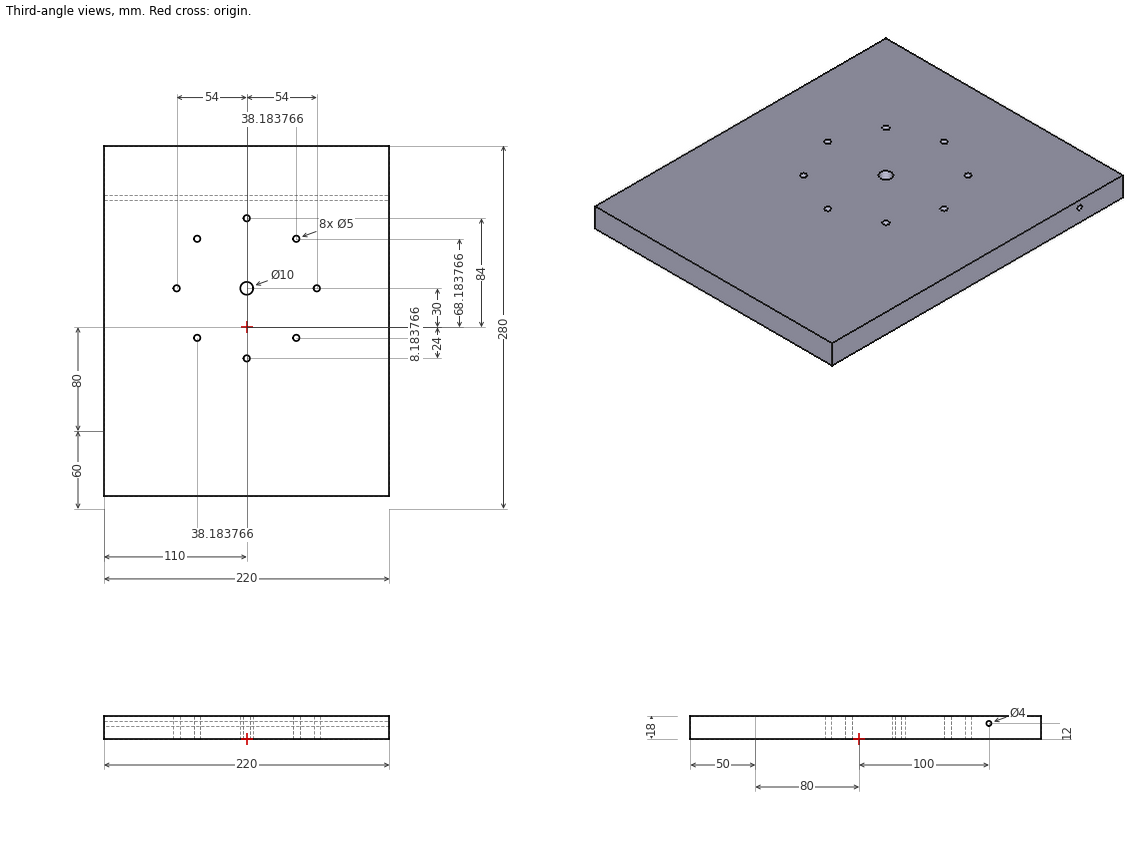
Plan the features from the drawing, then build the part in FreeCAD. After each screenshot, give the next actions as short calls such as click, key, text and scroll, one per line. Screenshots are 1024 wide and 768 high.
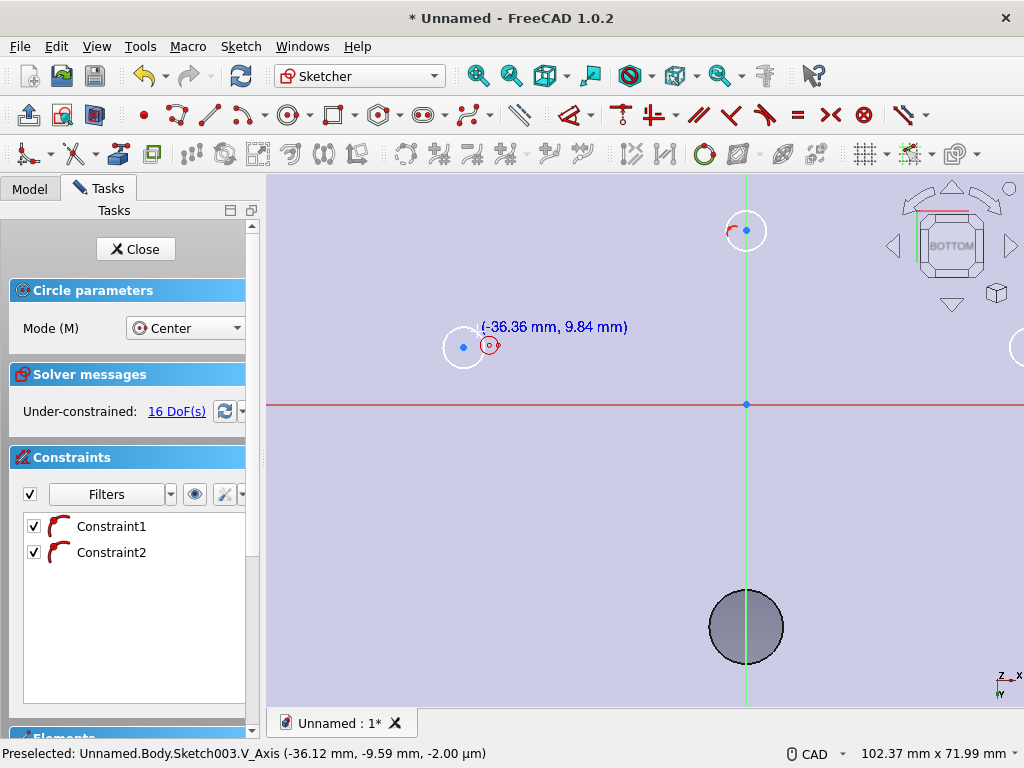
scroll(346, 627, up, 2)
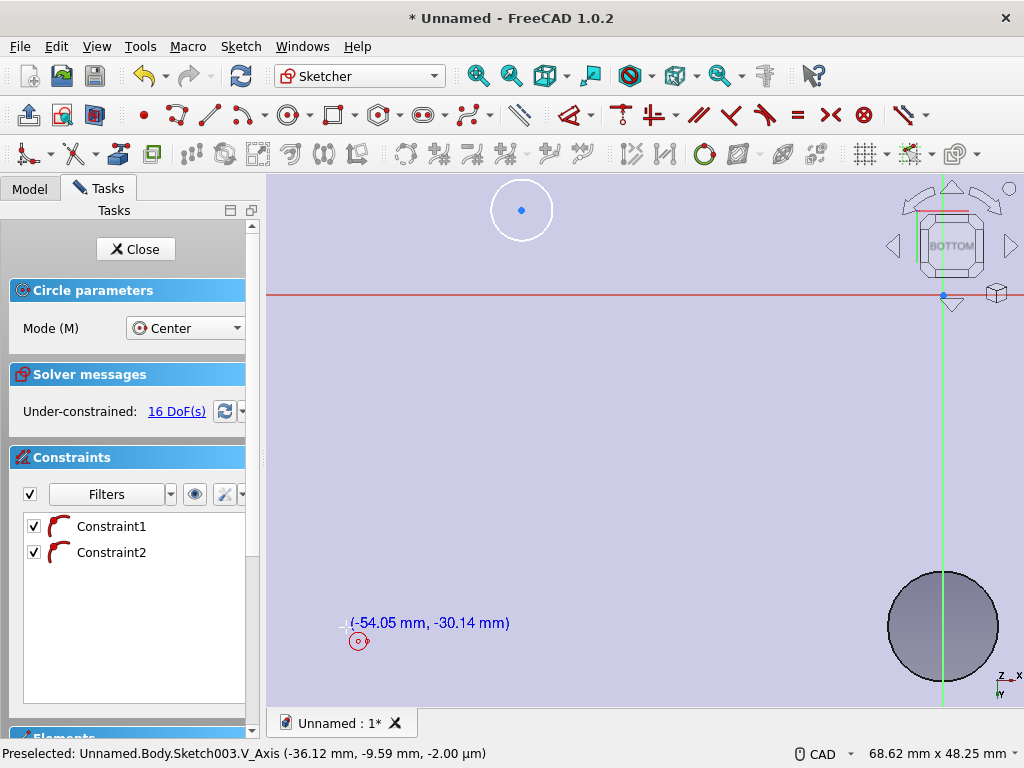
scroll(457, 380, down, 7)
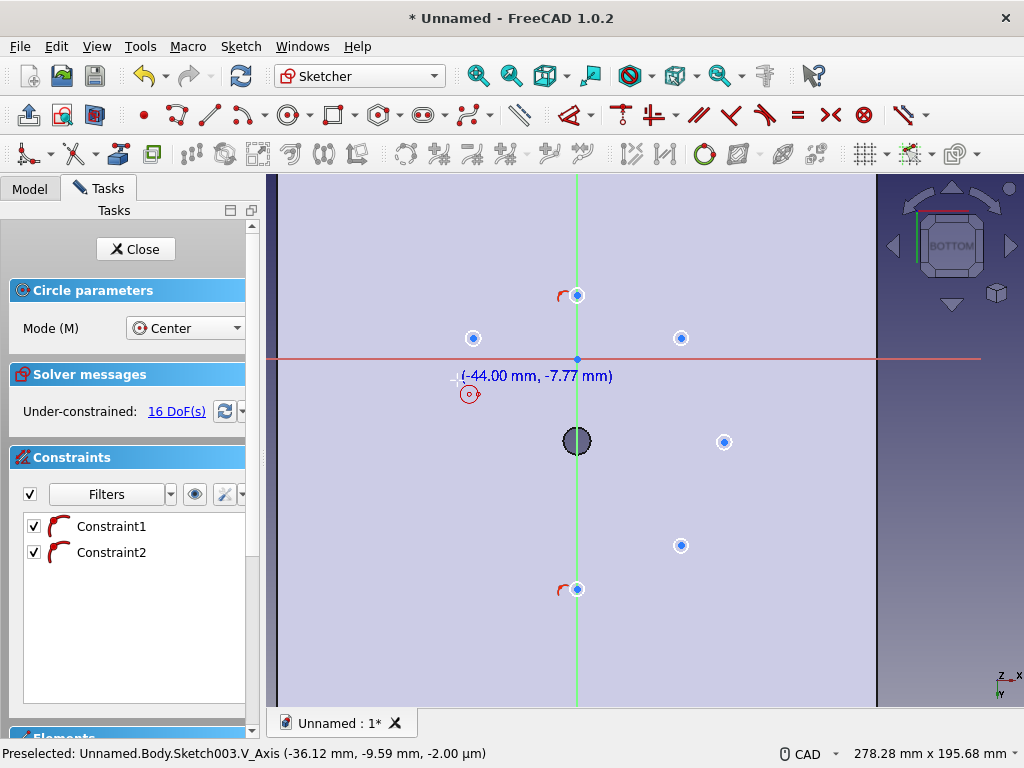
click(430, 441)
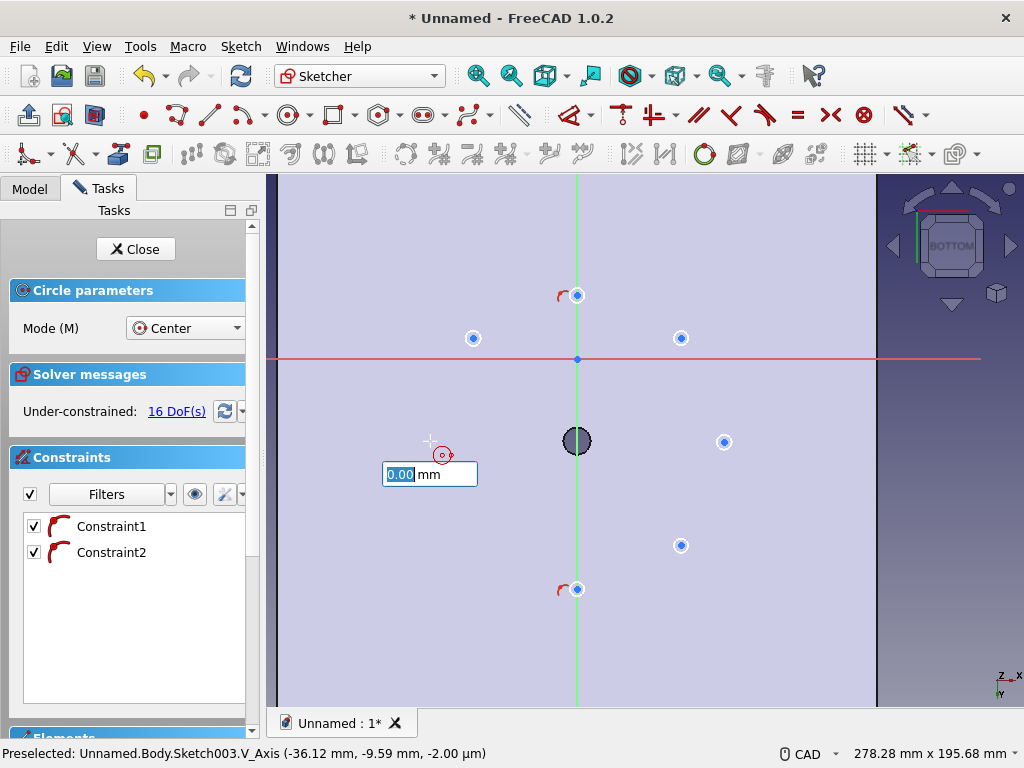
scroll(435, 436, up, 5)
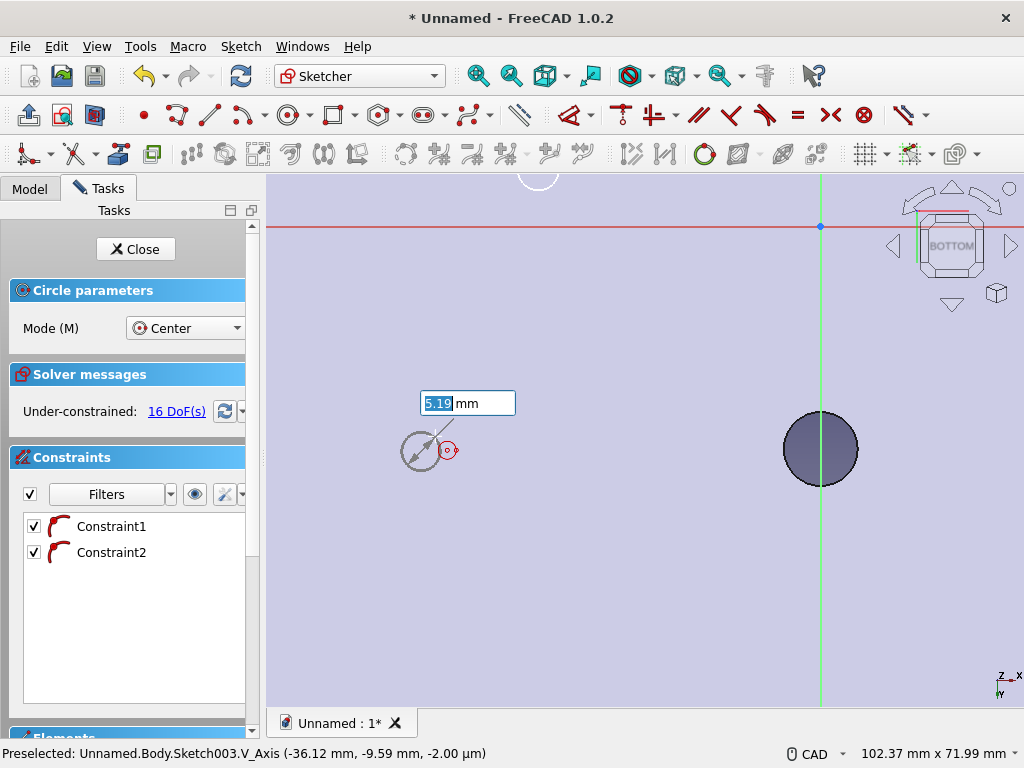
click(434, 436)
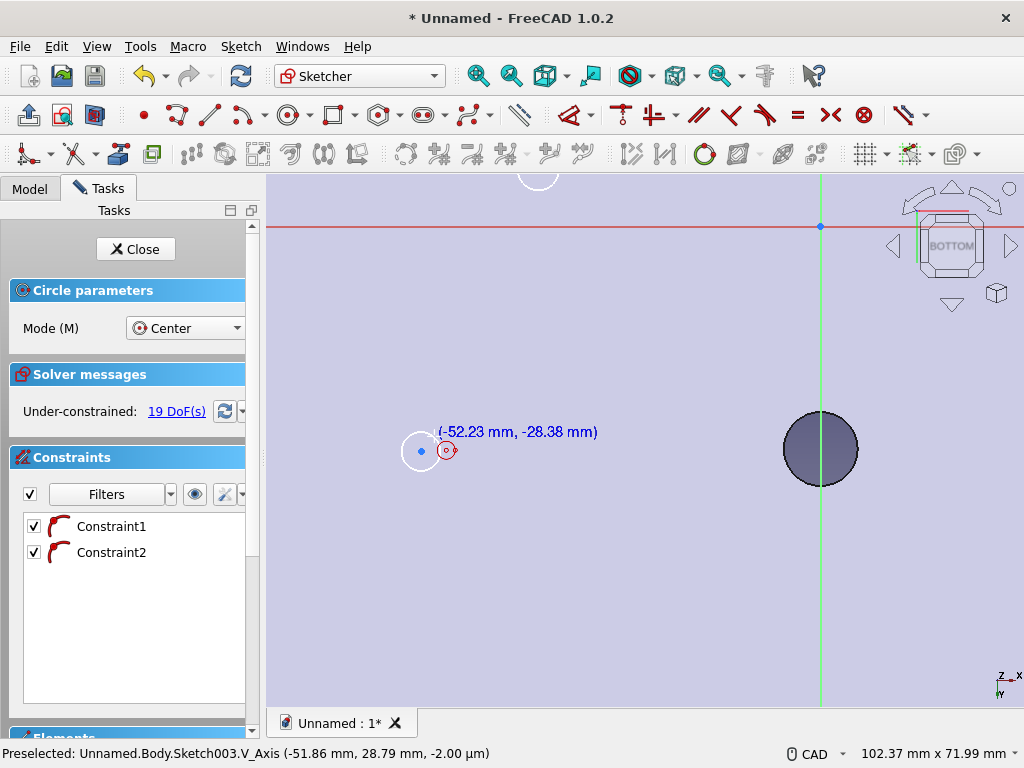
scroll(434, 436, down, 5)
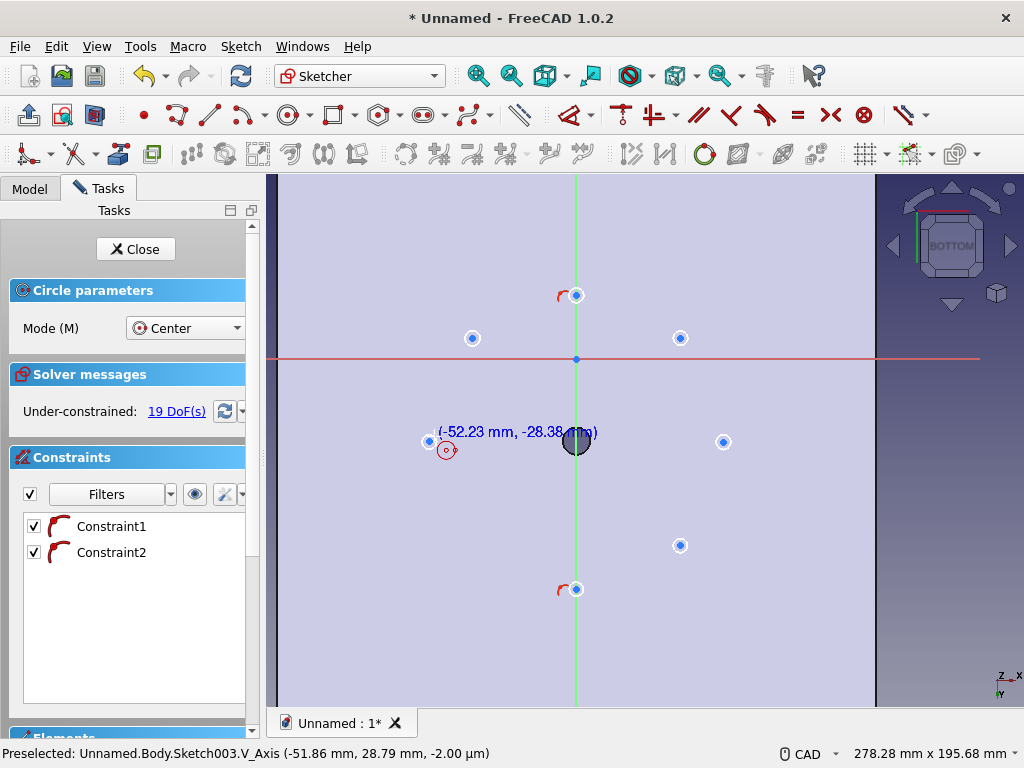
scroll(472, 545, up, 7)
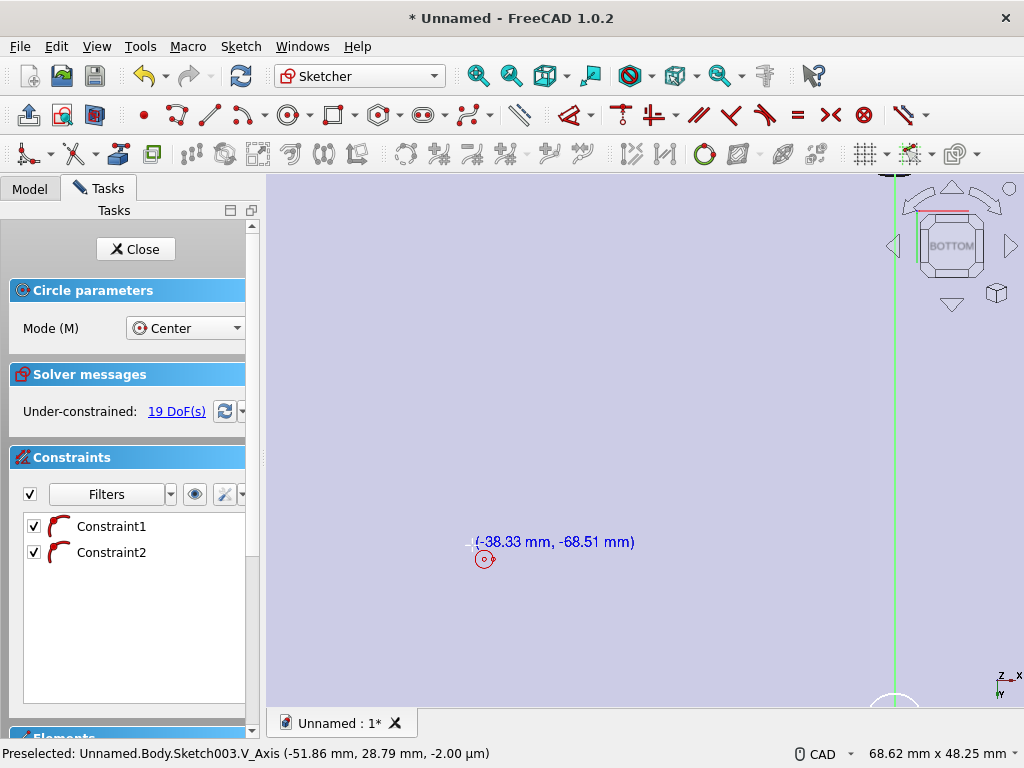
scroll(472, 545, down, 7)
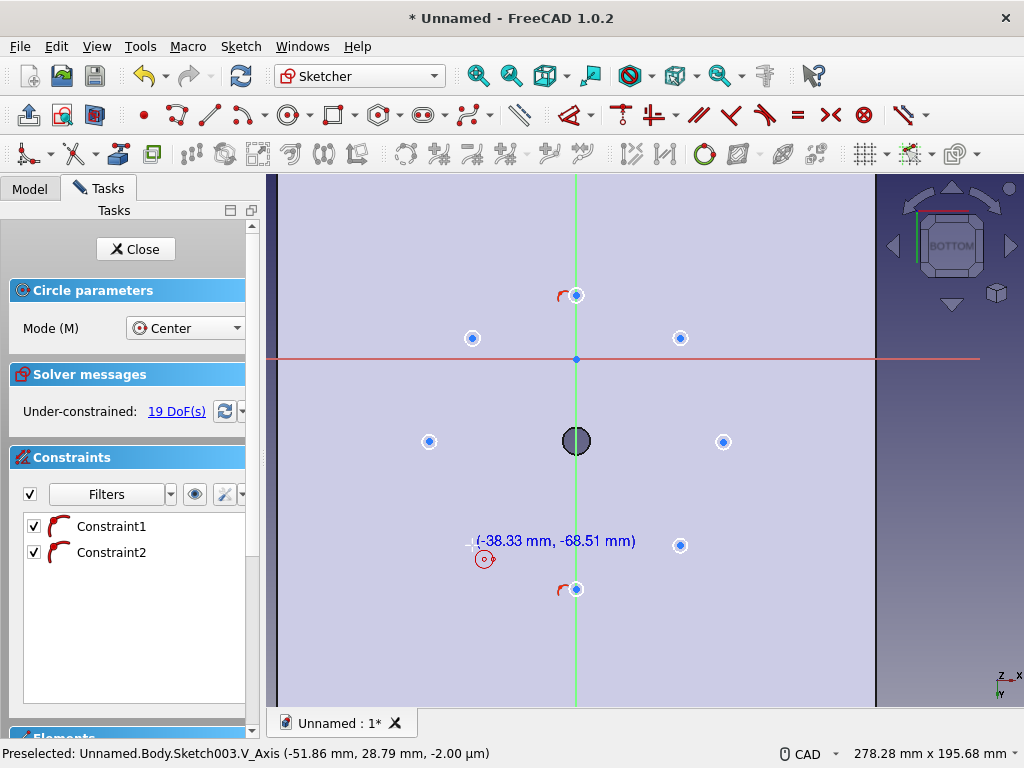
click(472, 545)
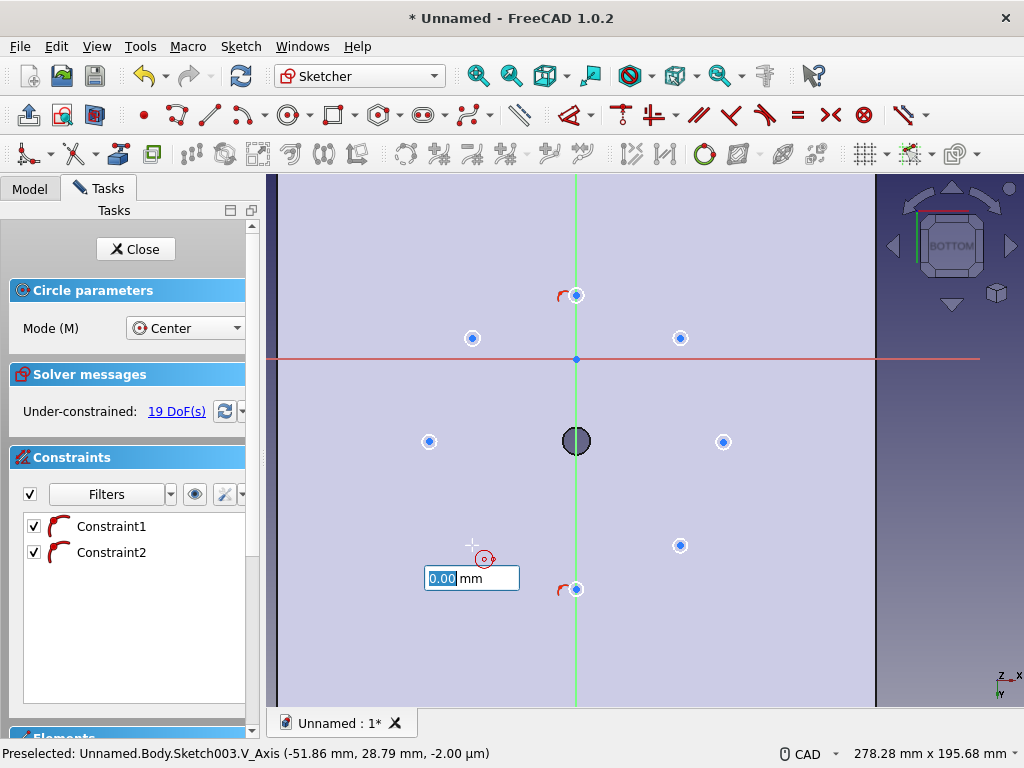
scroll(477, 540, up, 5)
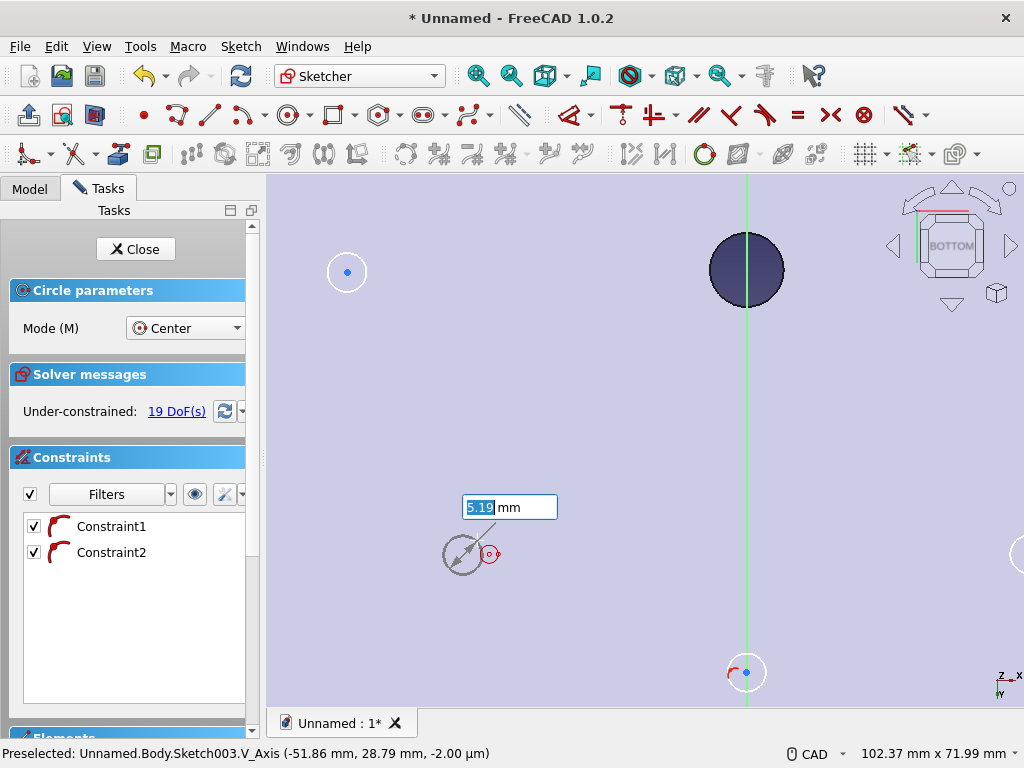
click(477, 540)
key(Escape)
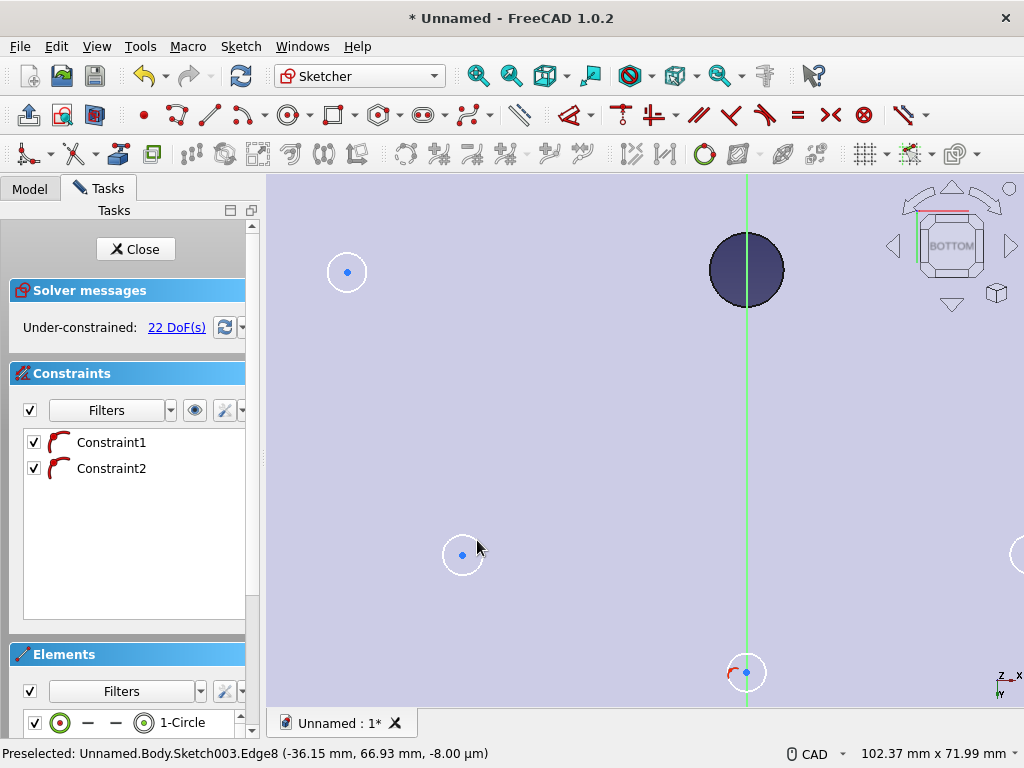
scroll(477, 540, down, 5)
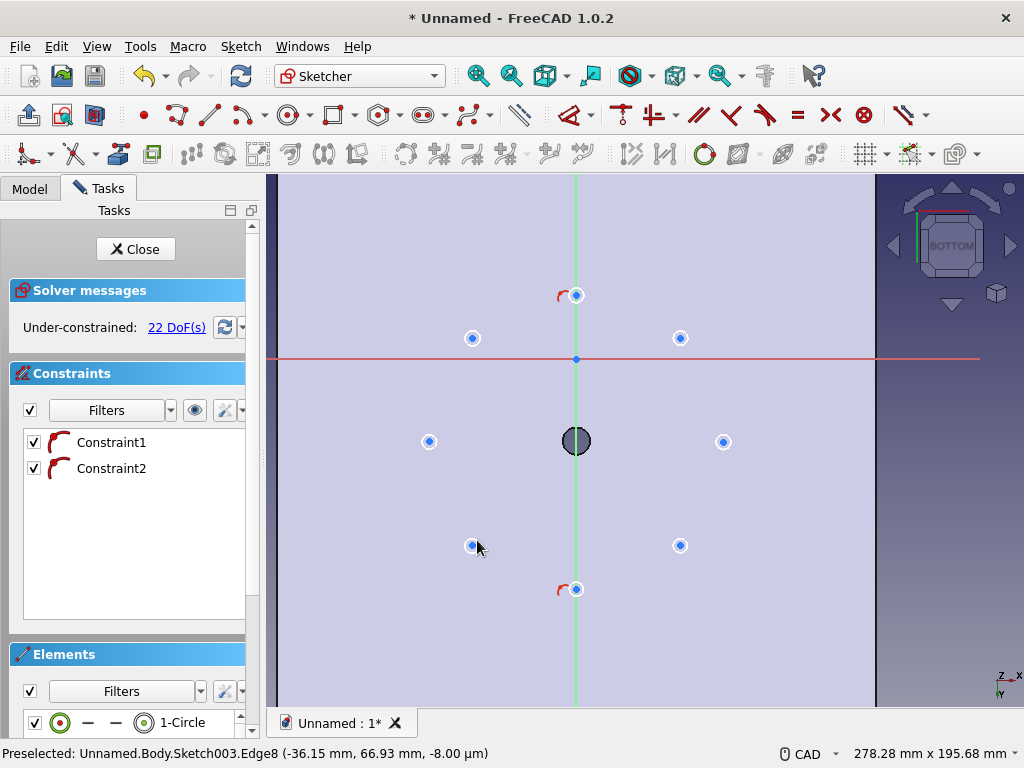
scroll(685, 541, up, 4)